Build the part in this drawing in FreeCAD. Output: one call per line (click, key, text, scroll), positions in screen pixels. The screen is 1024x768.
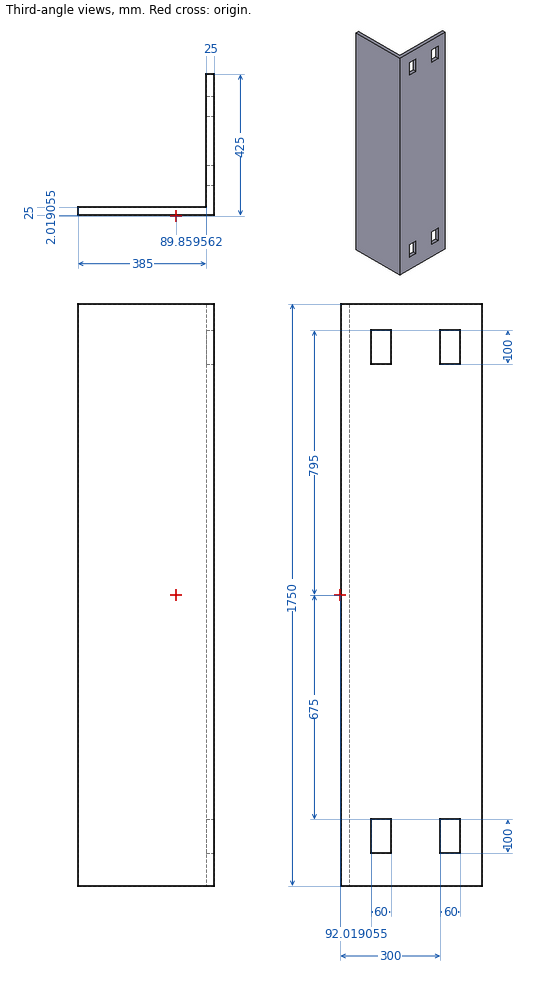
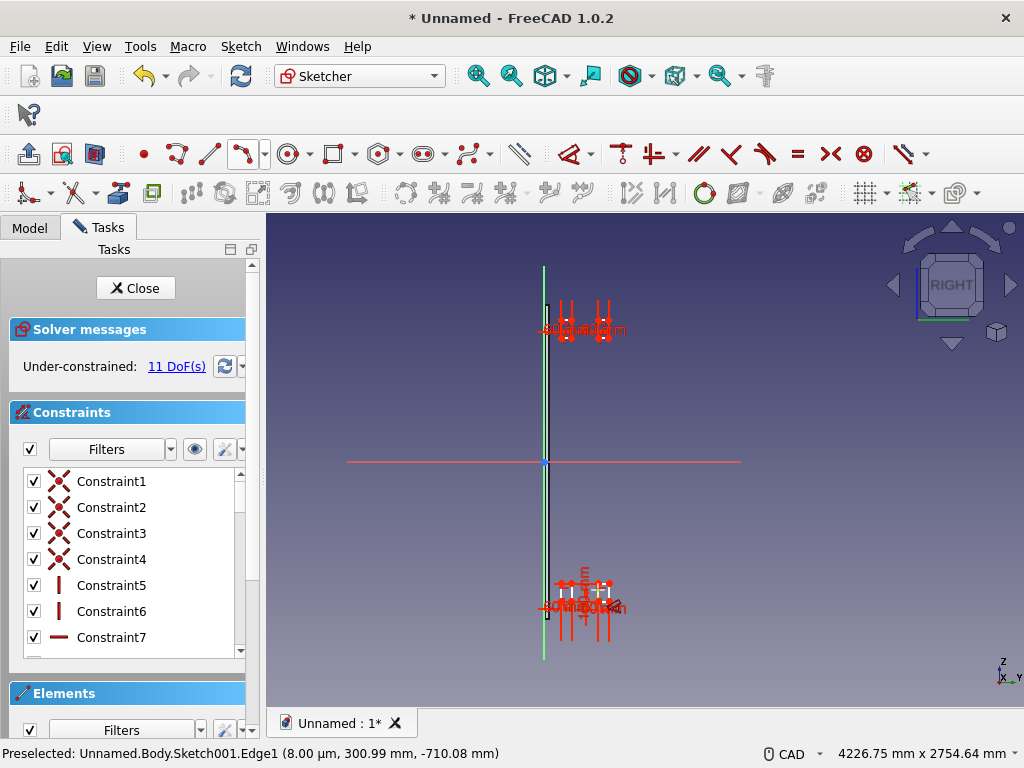
scroll(598, 326, up, 5)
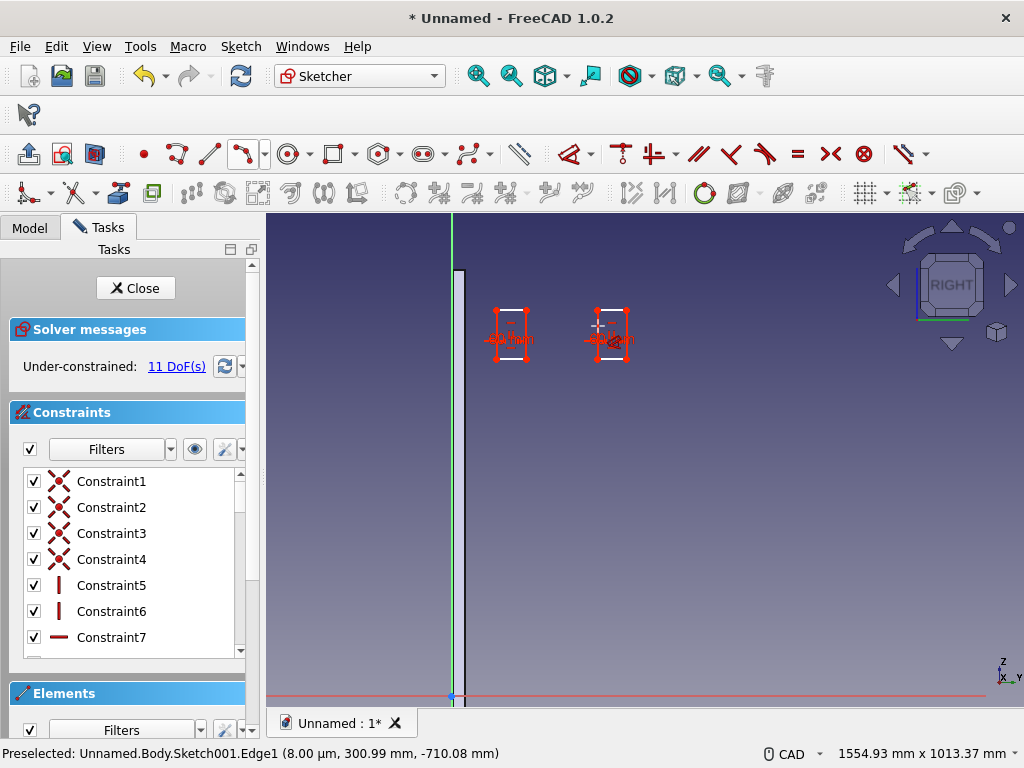
click(598, 325)
click(564, 318)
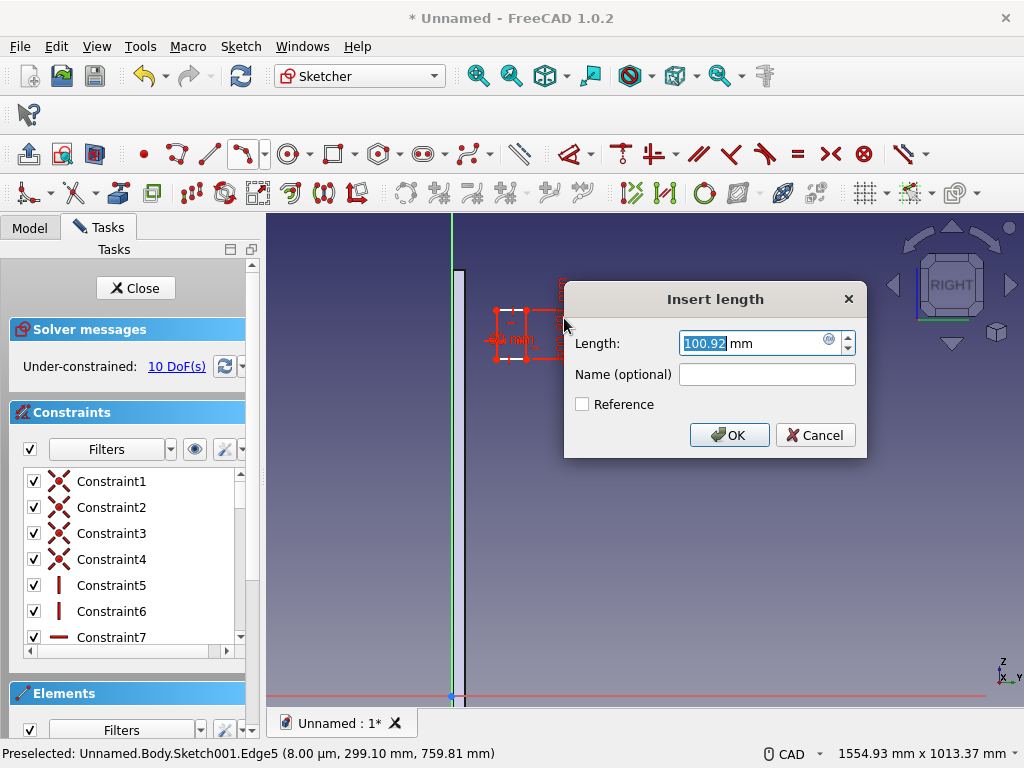
text(100)
key(Return)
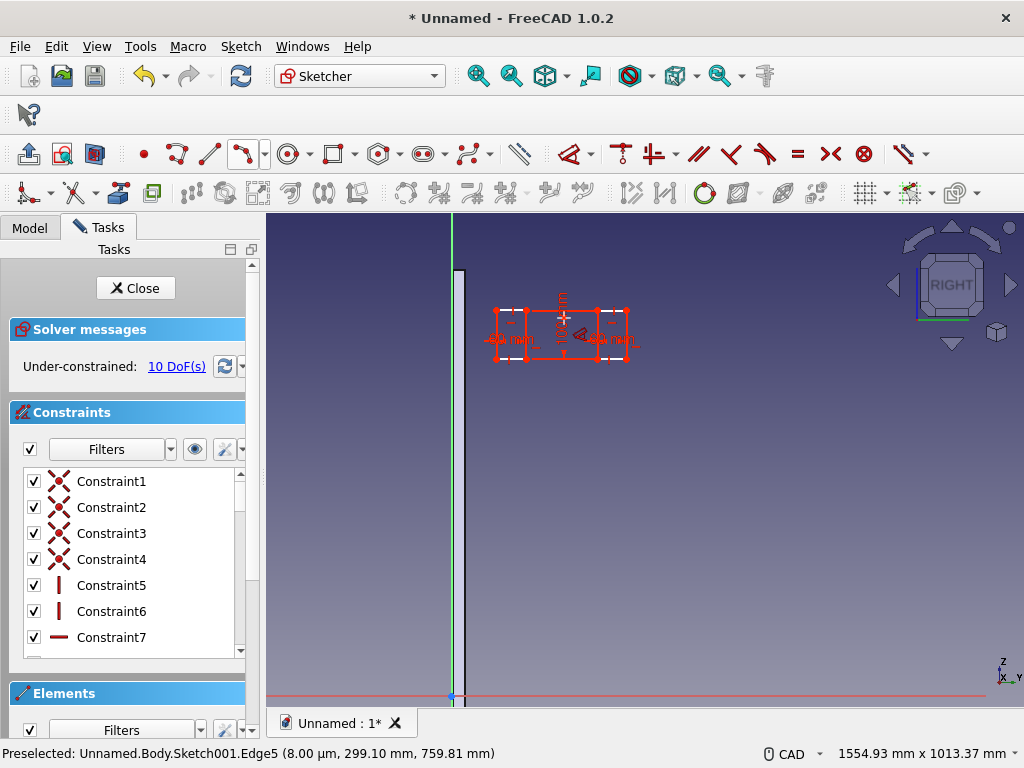
scroll(598, 325, down, 5)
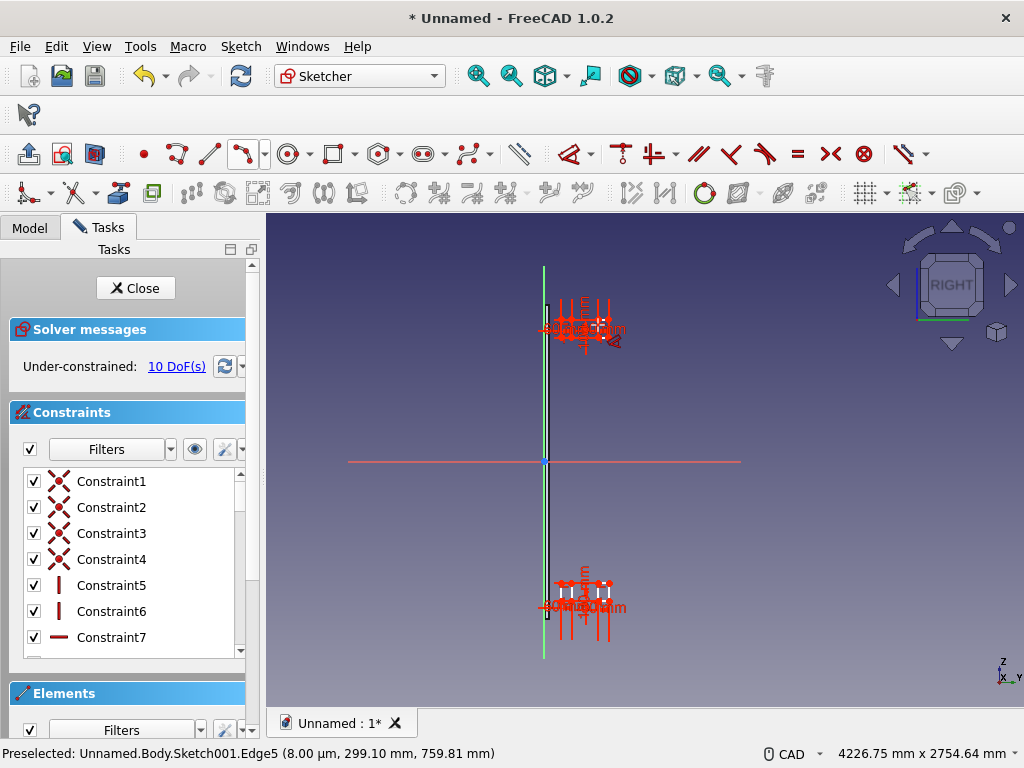
scroll(561, 589, up, 5)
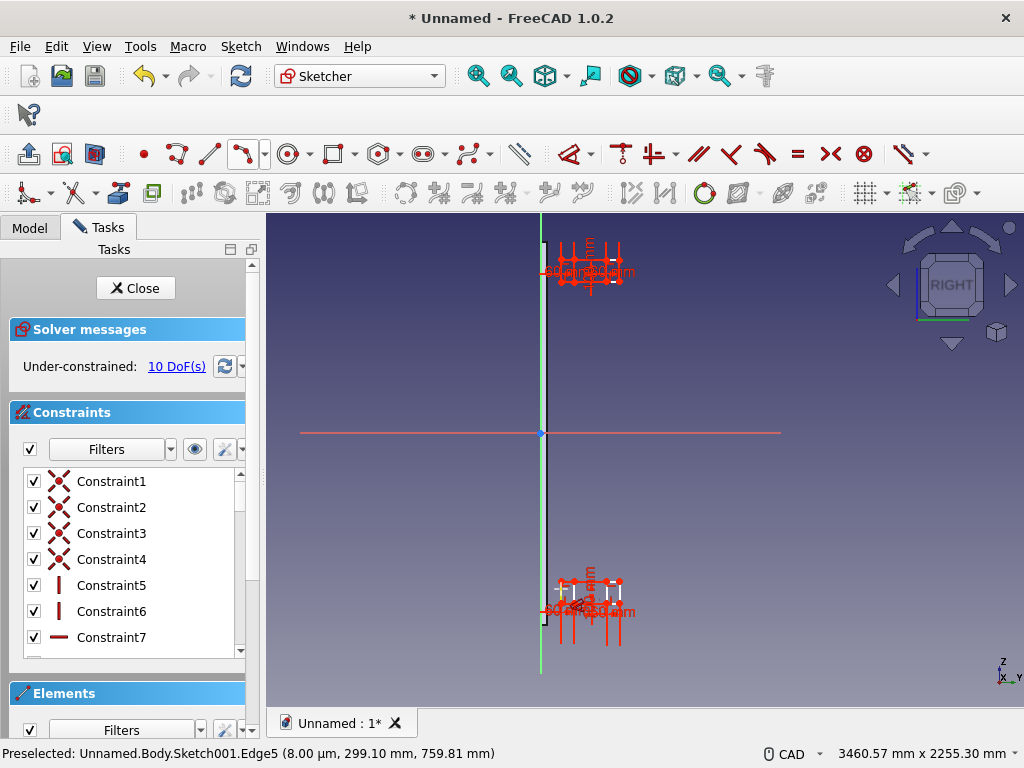
click(561, 587)
click(479, 597)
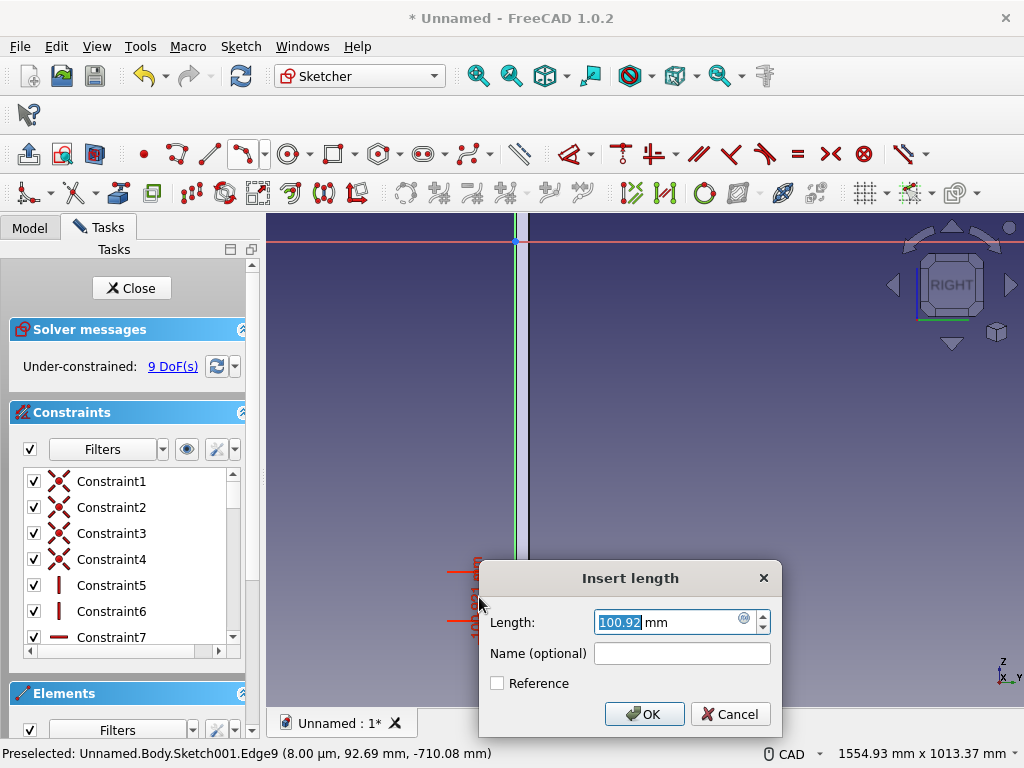
text(100)
key(Return)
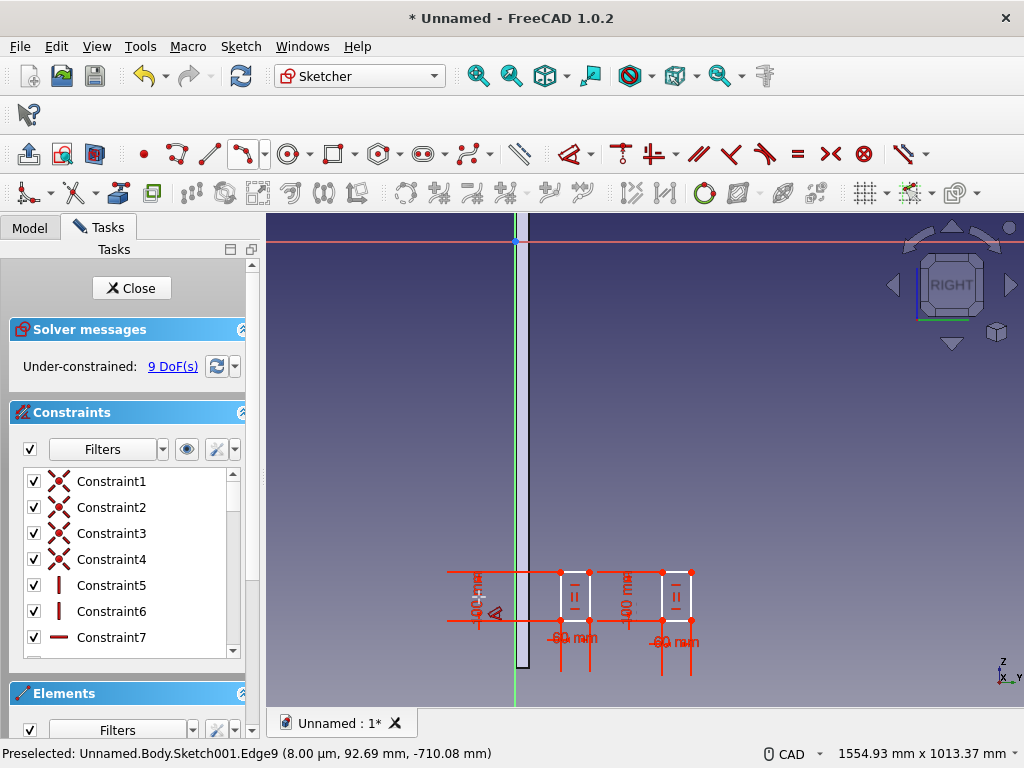
scroll(561, 590, down, 5)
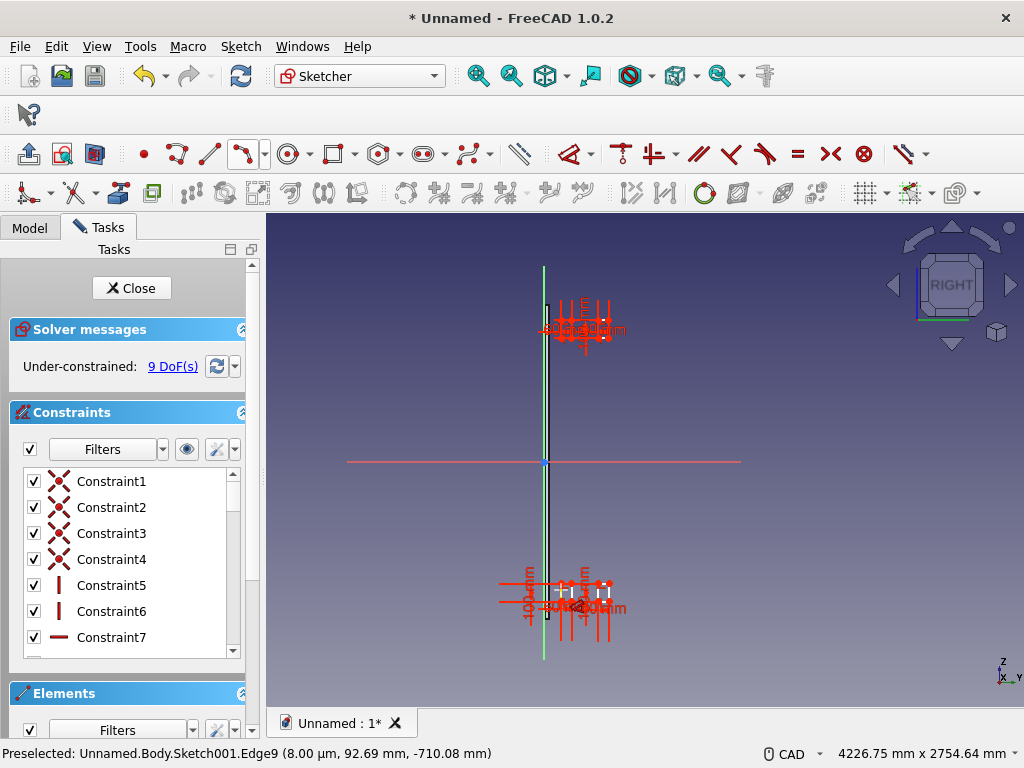
scroll(561, 326, up, 5)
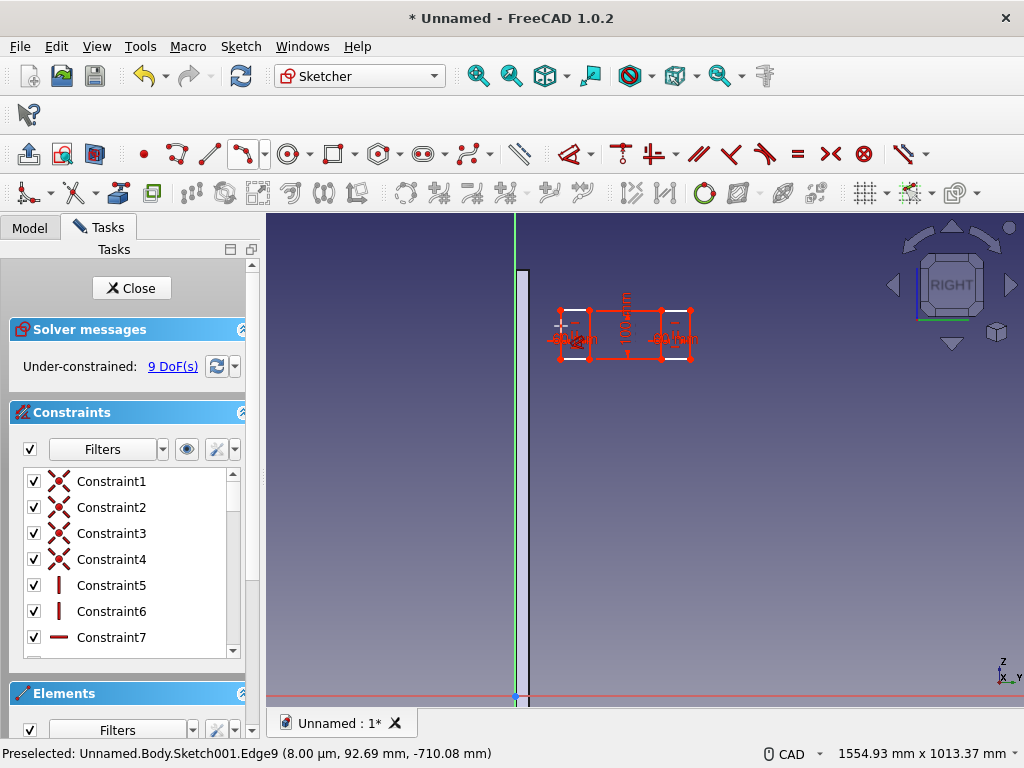
click(561, 325)
click(479, 335)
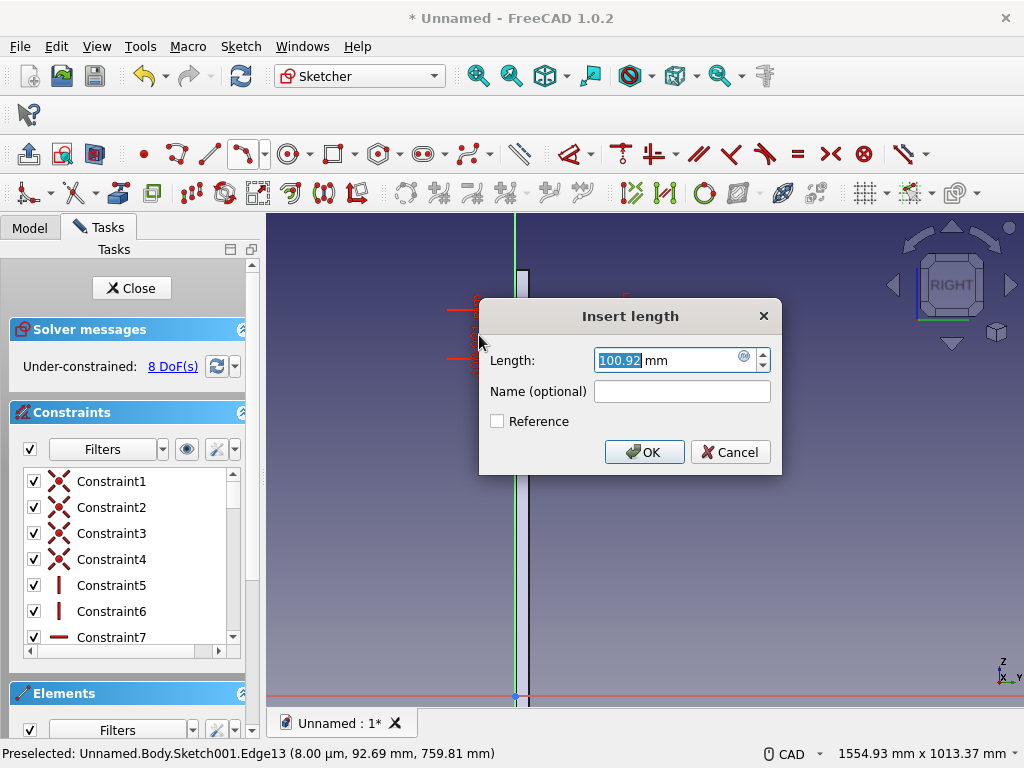
text(100)
key(Return)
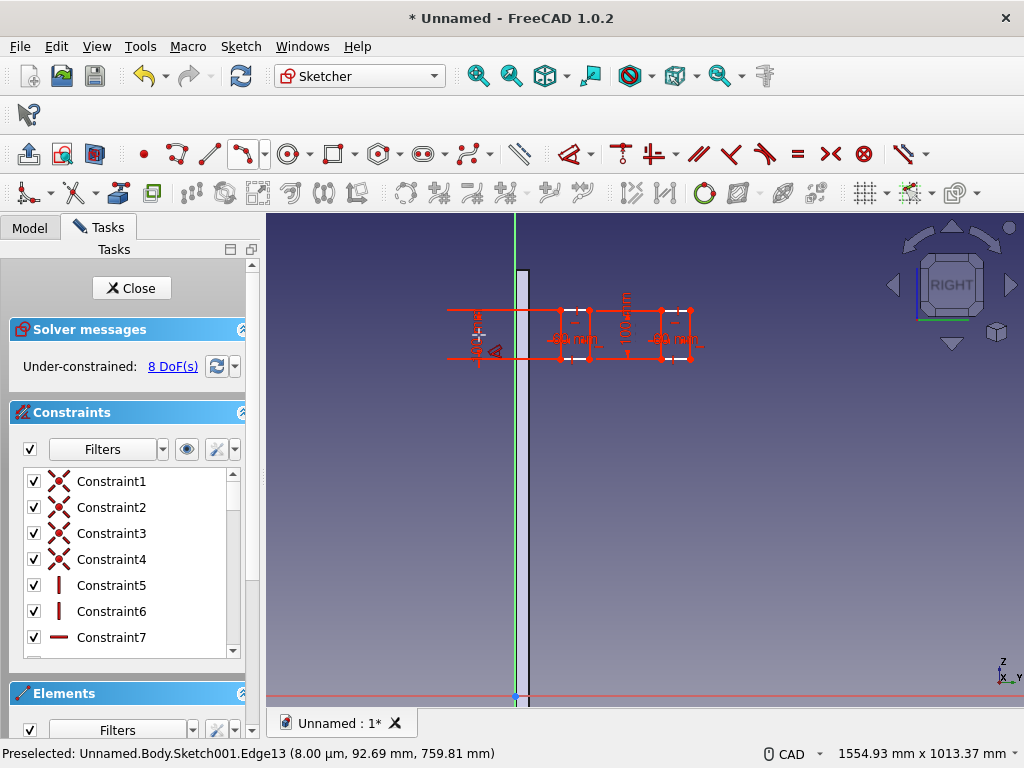
scroll(561, 325, down, 5)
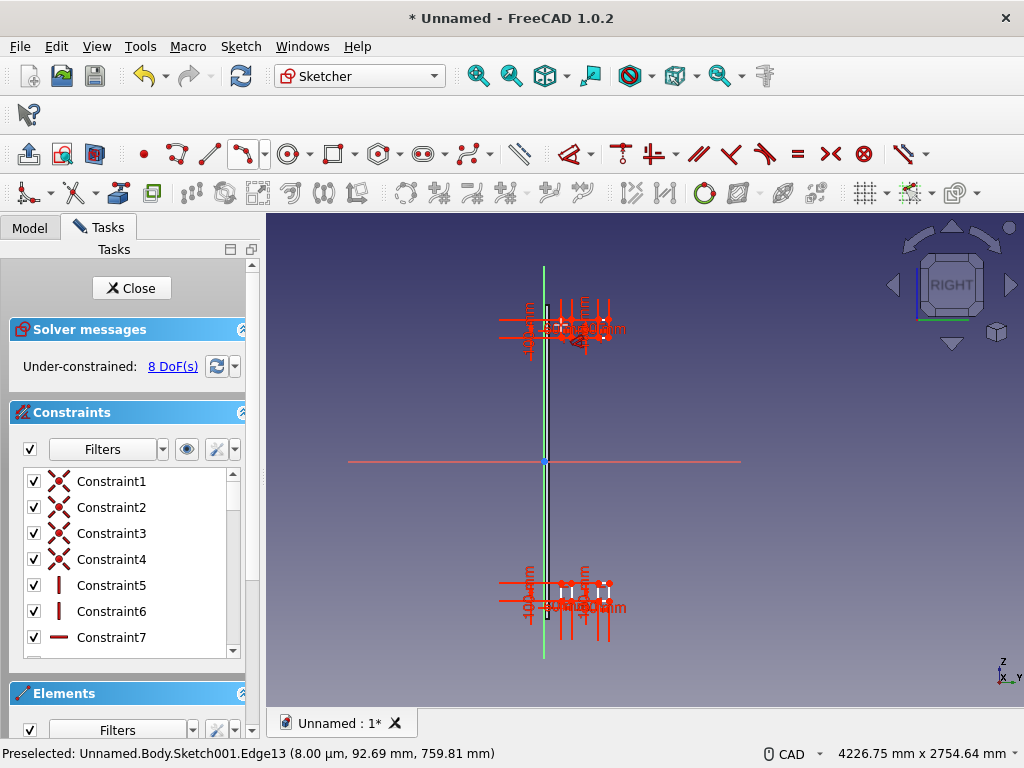
click(598, 583)
click(571, 428)